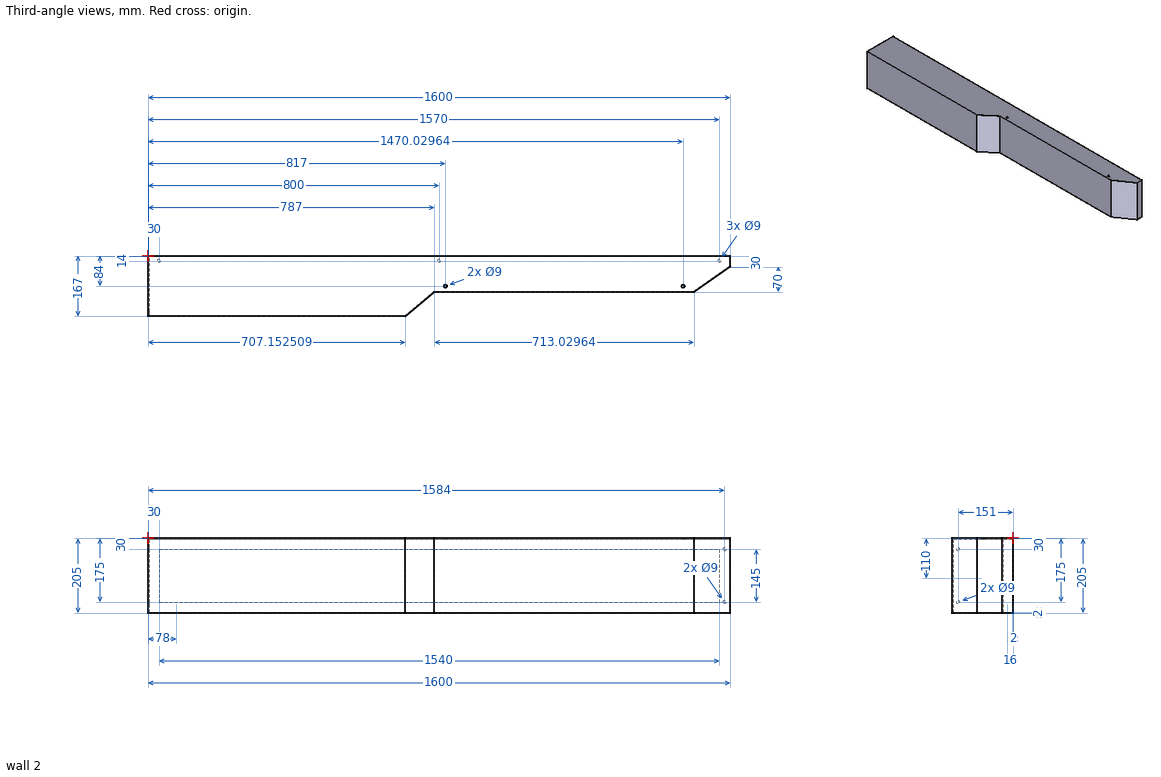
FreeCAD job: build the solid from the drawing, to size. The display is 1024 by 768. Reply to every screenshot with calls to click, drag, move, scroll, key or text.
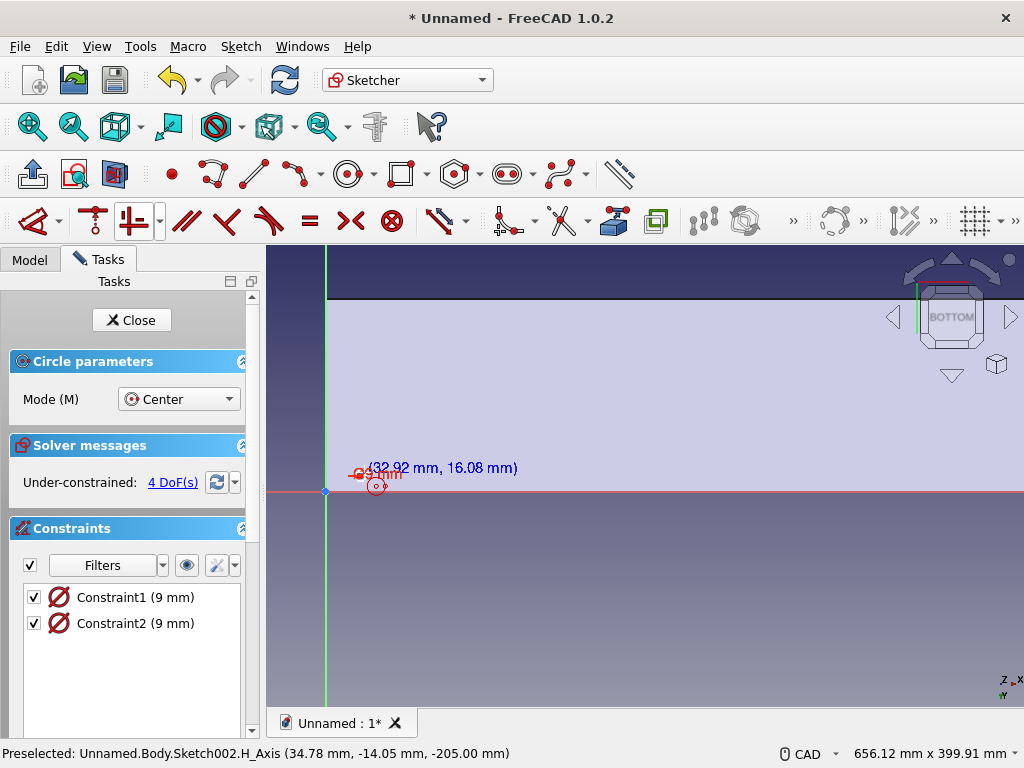
scroll(410, 475, down, 8)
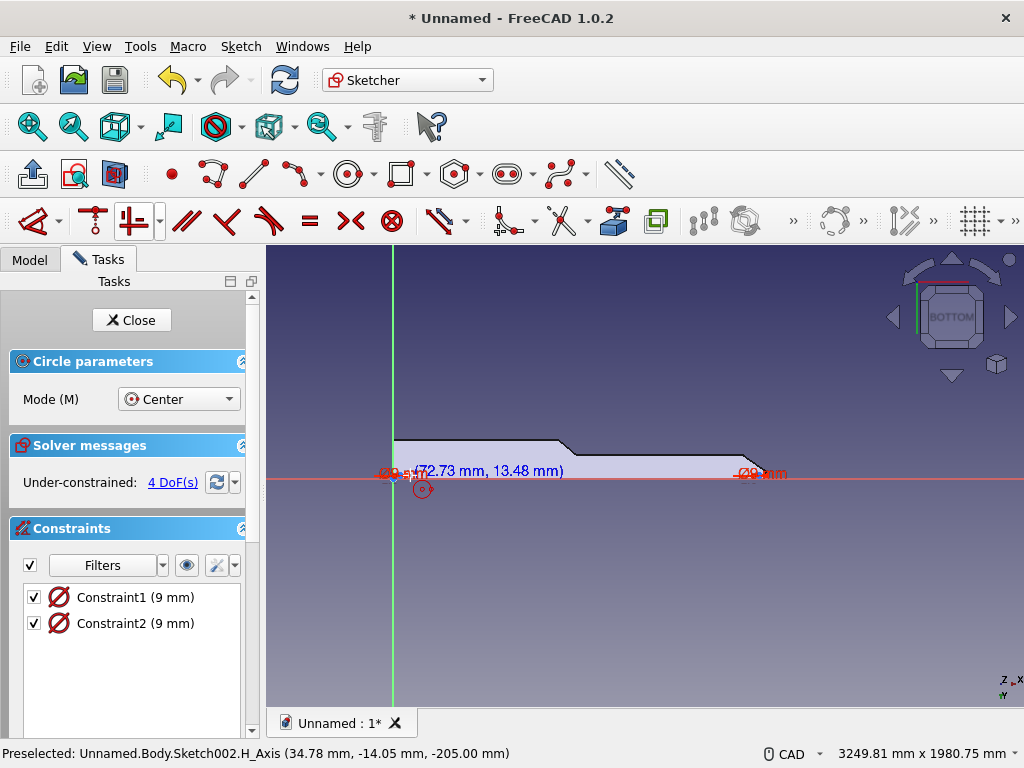
scroll(580, 475, up, 16)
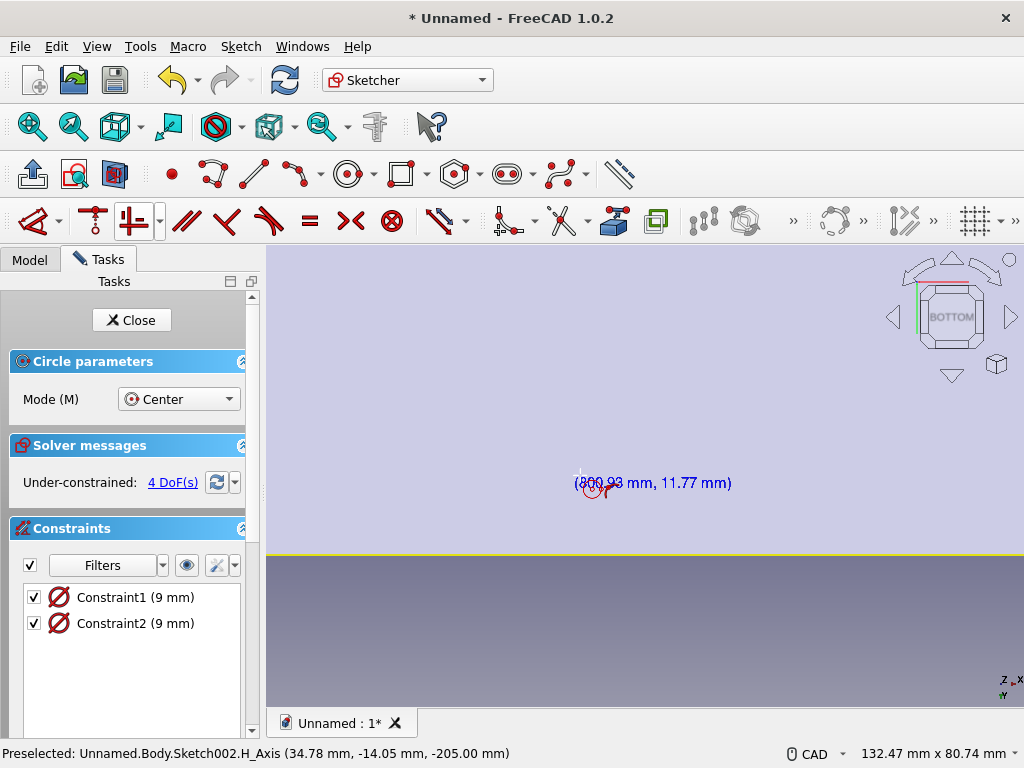
scroll(581, 475, down, 15)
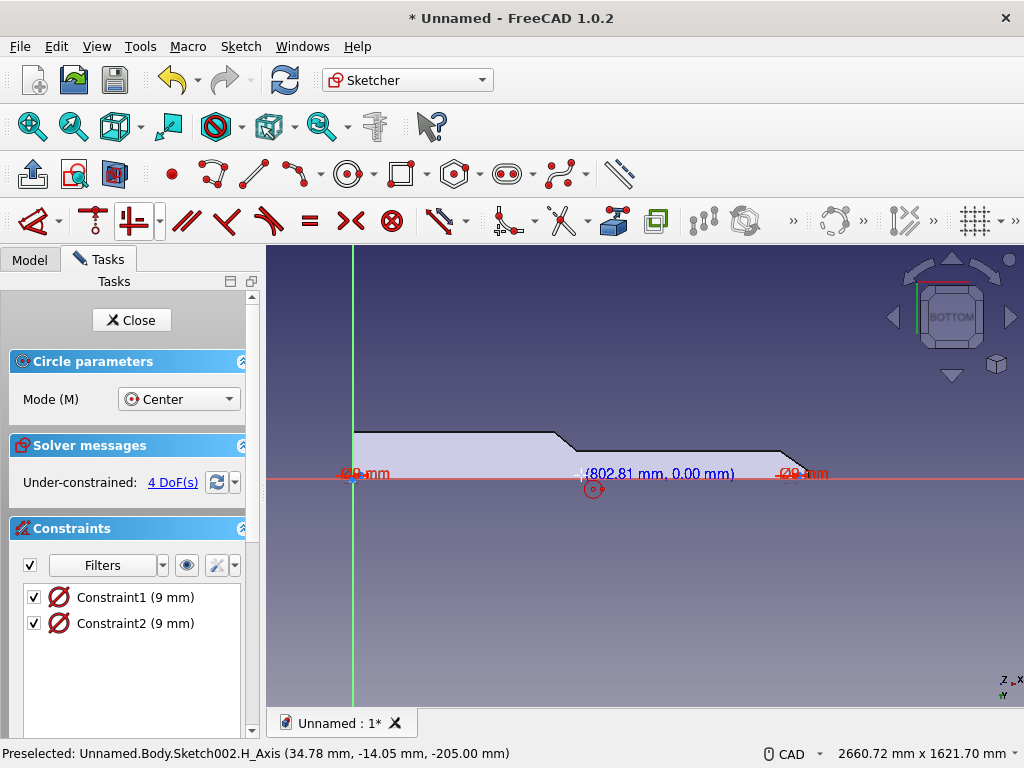
scroll(581, 475, up, 7)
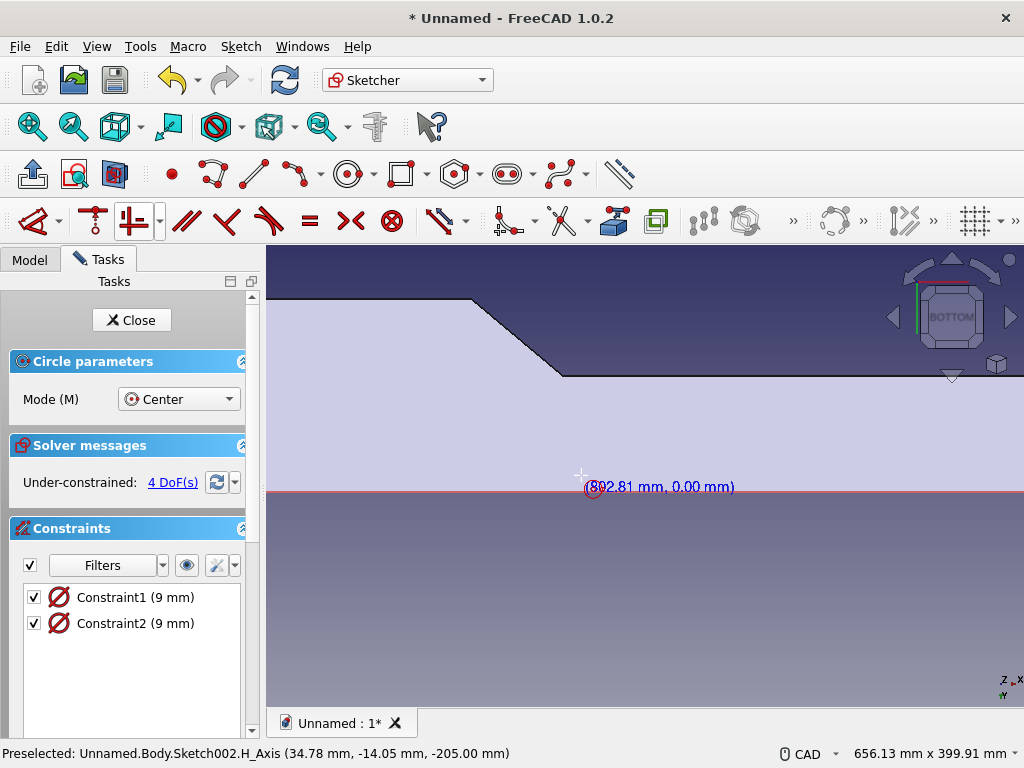
click(578, 475)
move(582, 472)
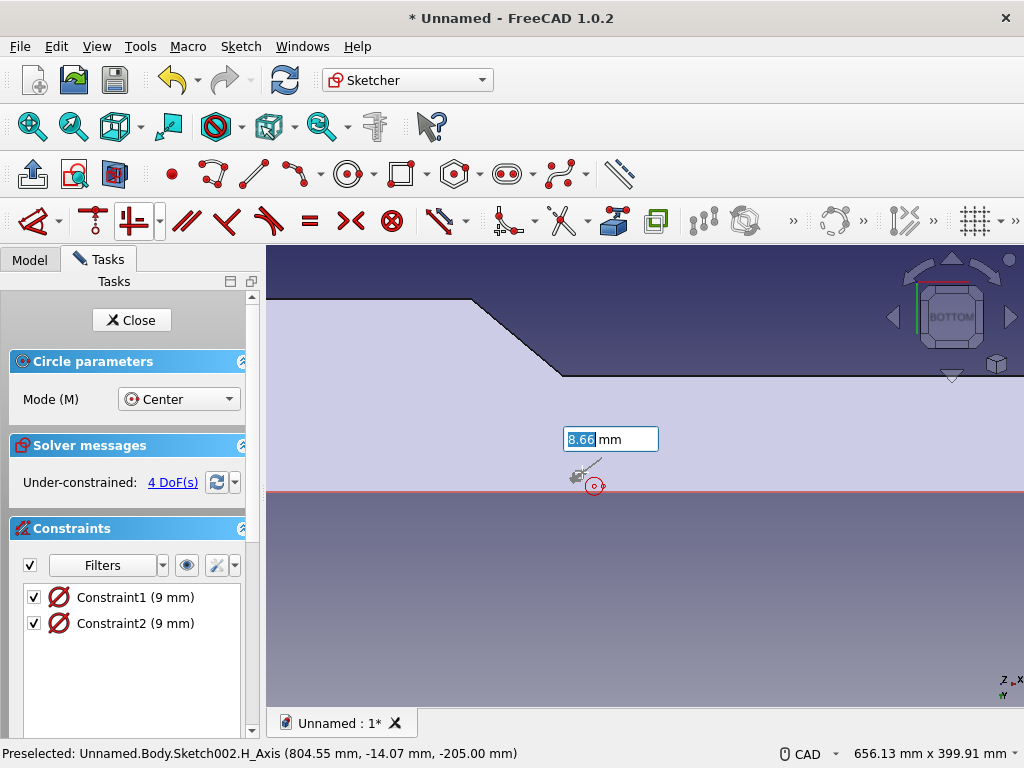
text(9)
key(Return)
key(Escape)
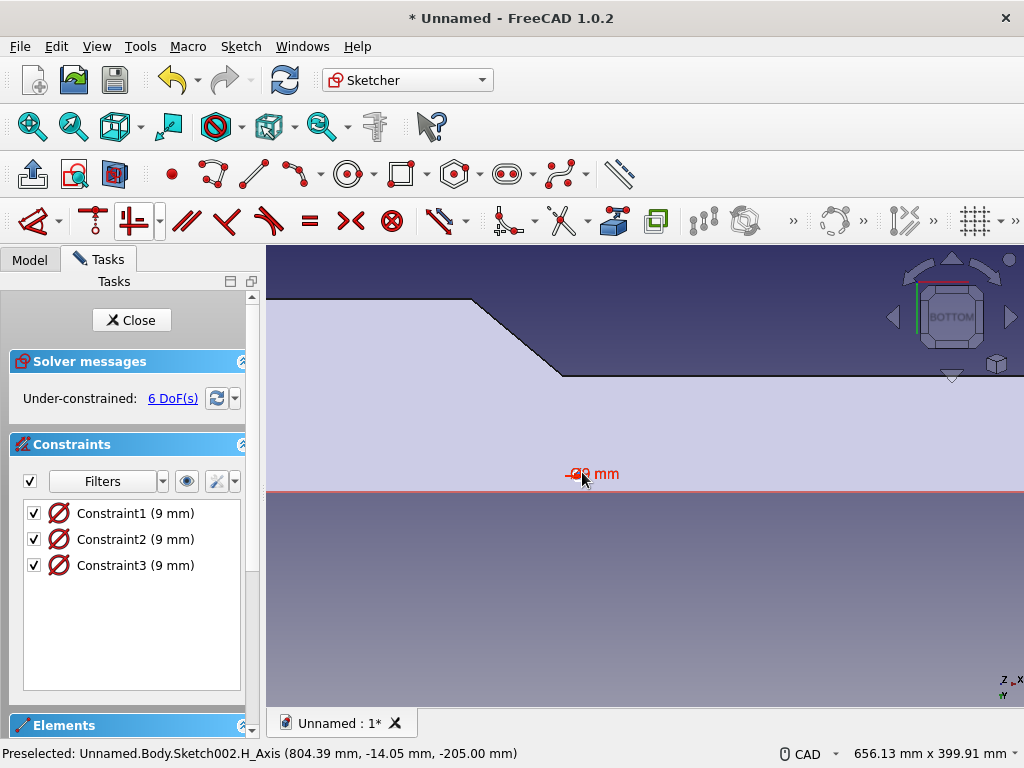
key(d)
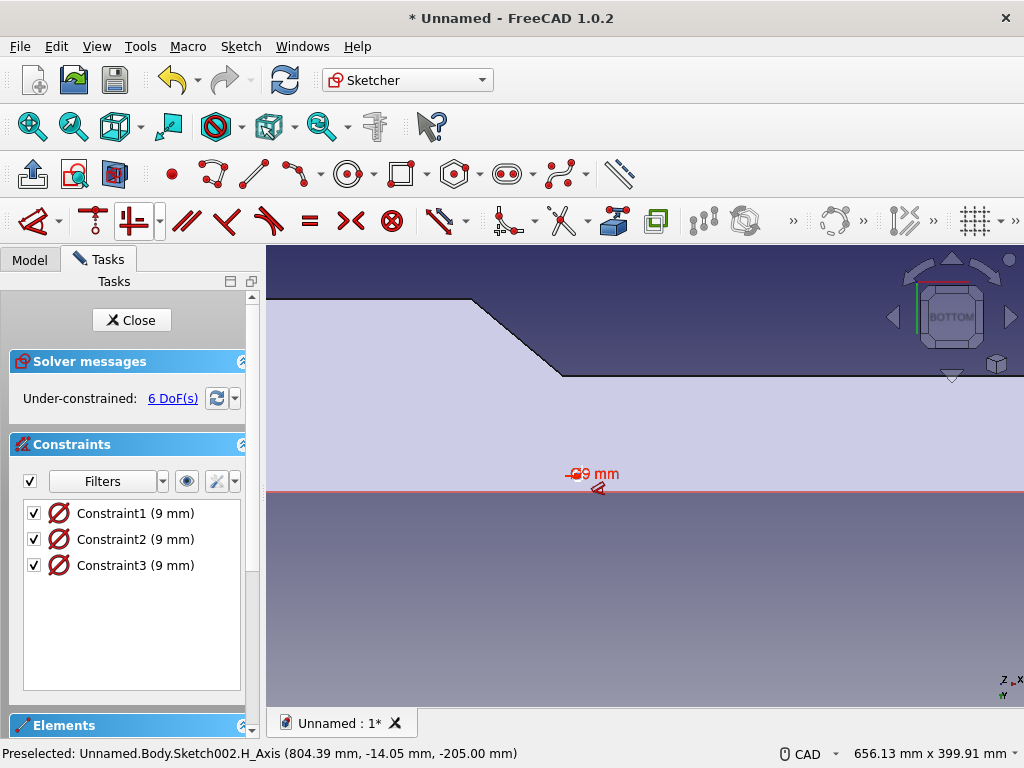
scroll(580, 475, down, 8)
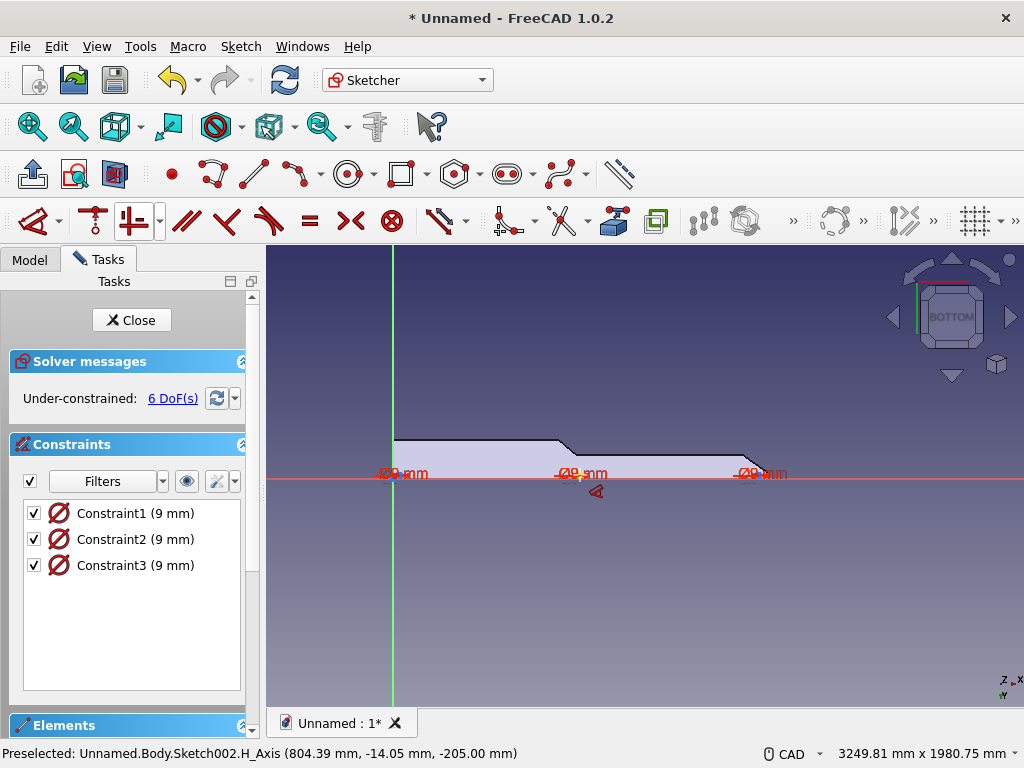
scroll(760, 476, up, 13)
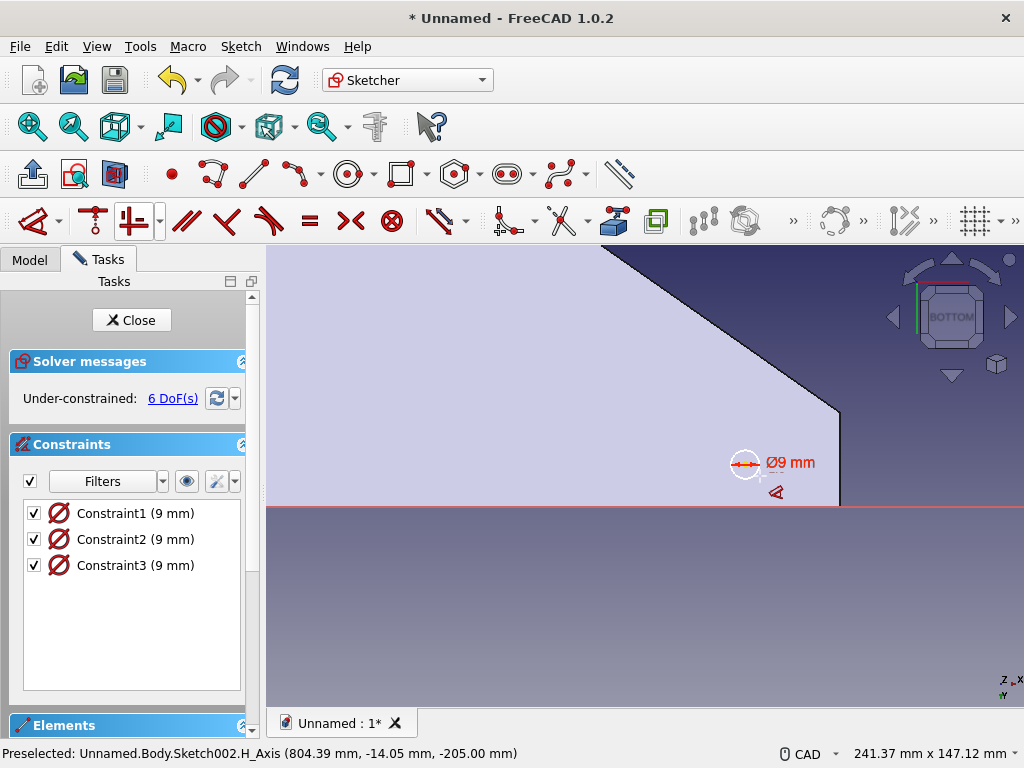
click(745, 465)
click(779, 486)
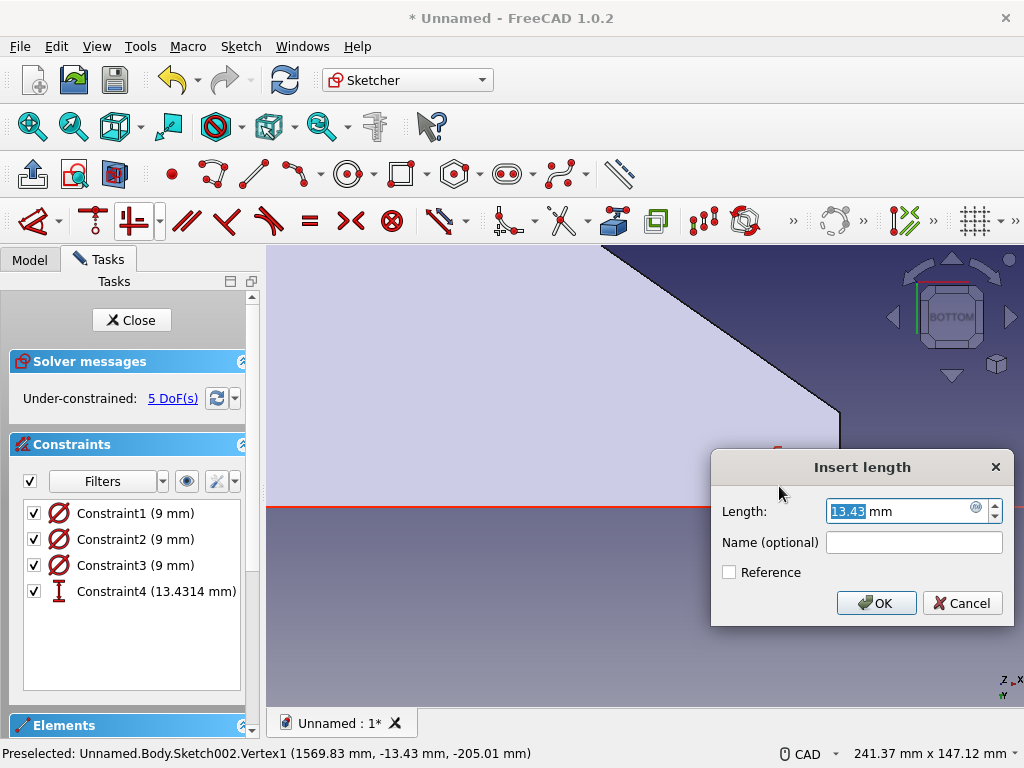
text(14)
key(Return)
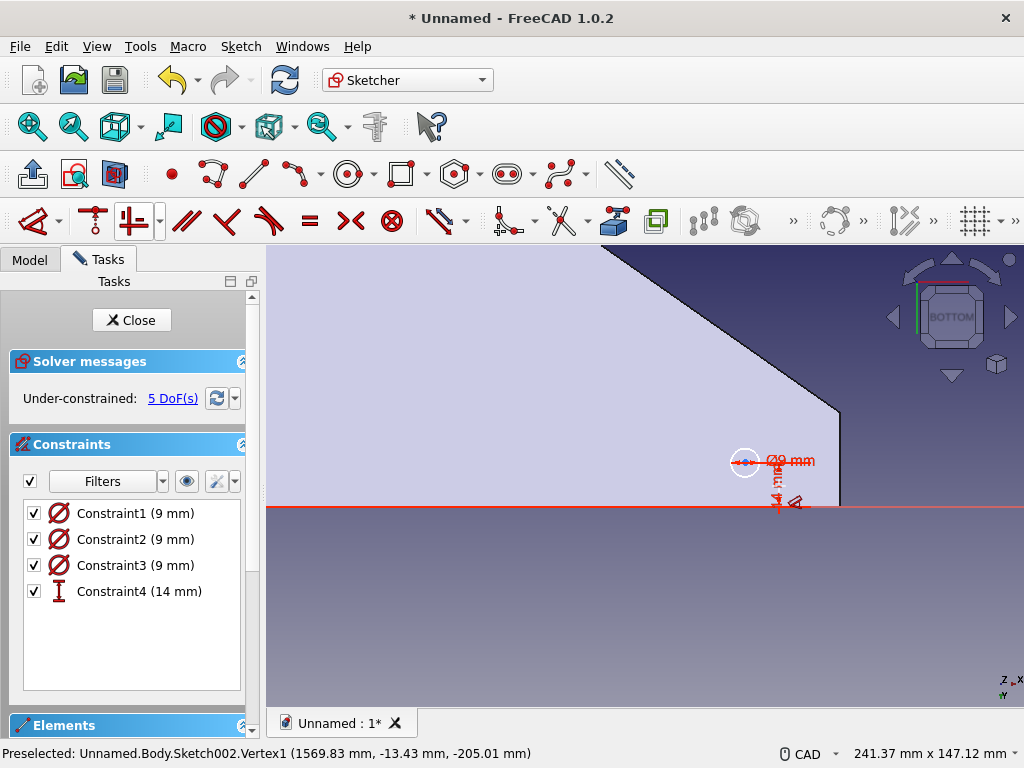
scroll(760, 476, down, 13)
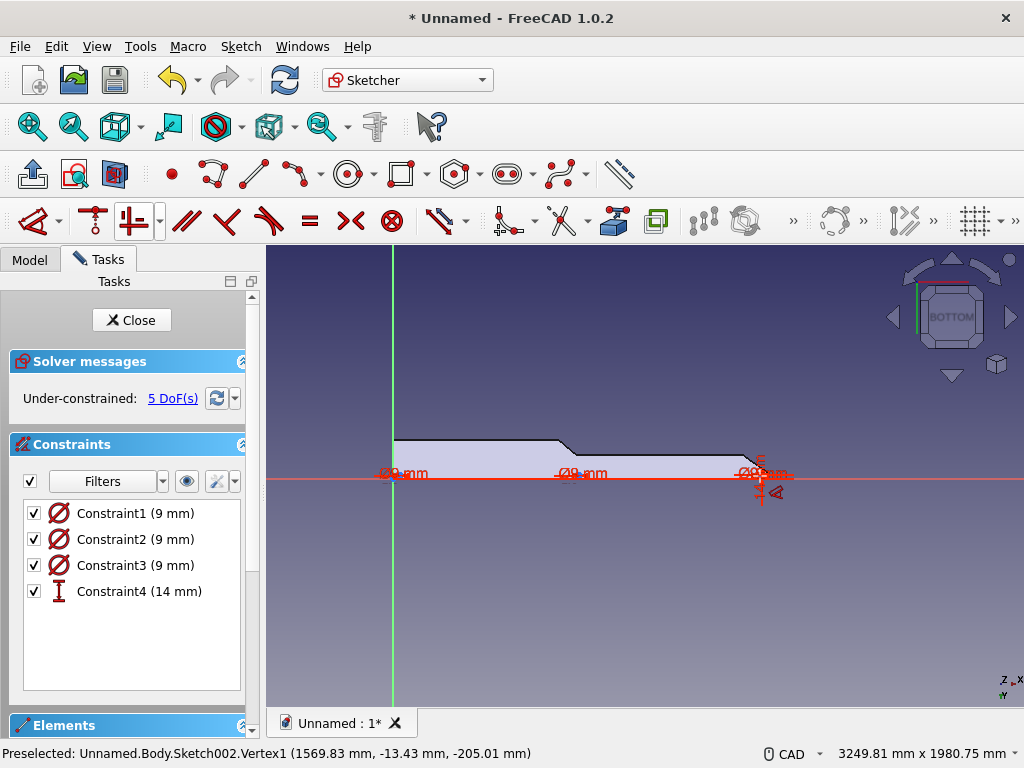
scroll(400, 476, up, 9)